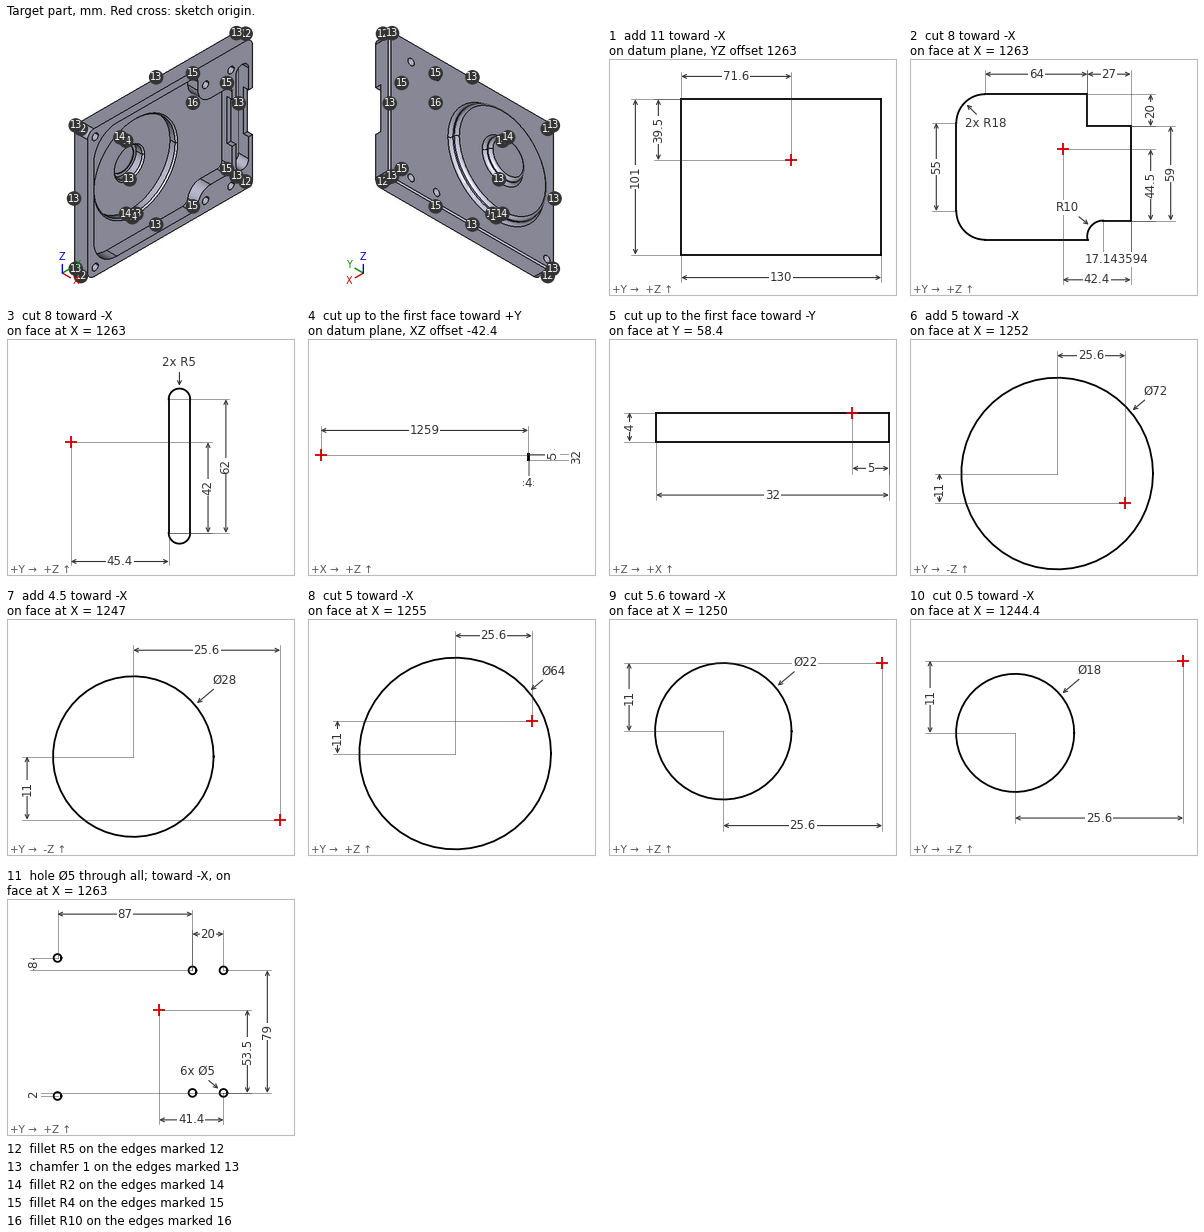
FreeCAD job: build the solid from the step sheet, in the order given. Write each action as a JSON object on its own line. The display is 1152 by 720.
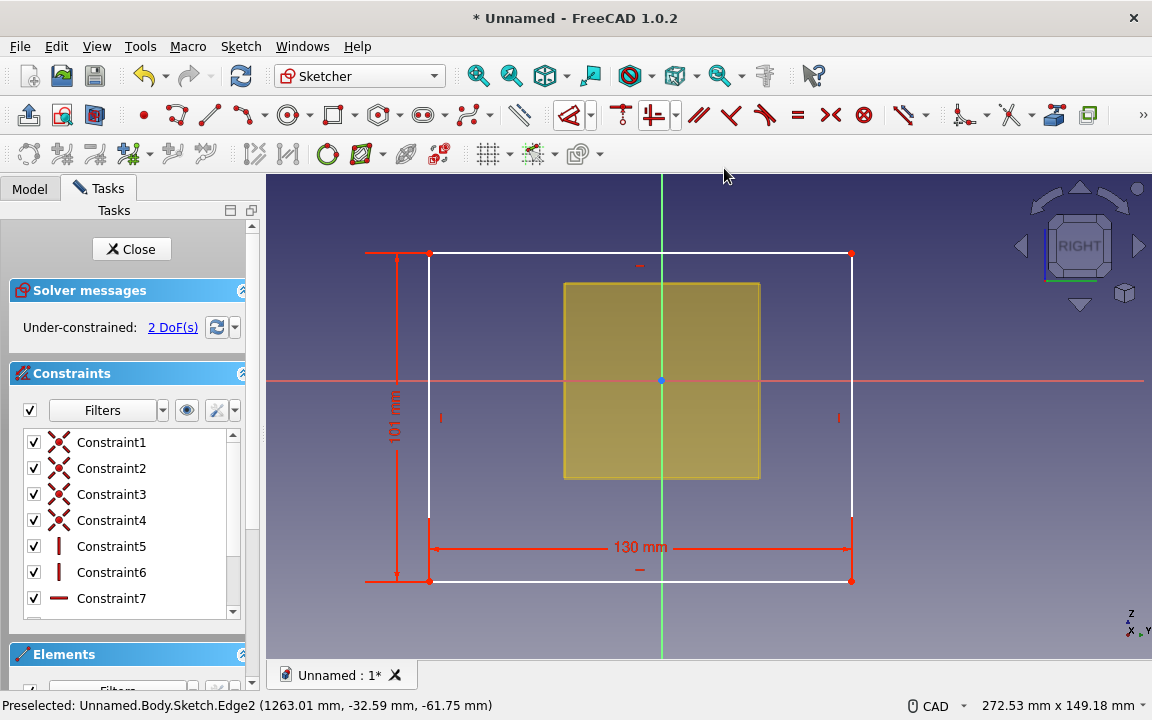
{"action": "left_click", "coordinate": [429, 253]}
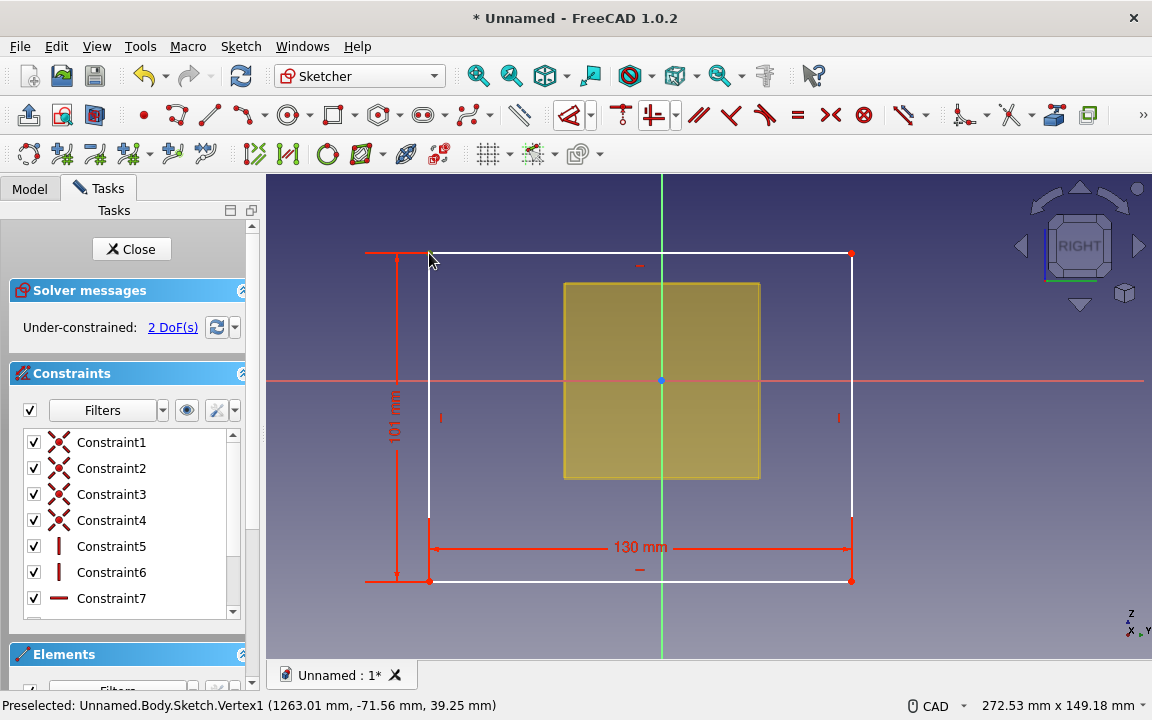
{"action": "key", "text": "l"}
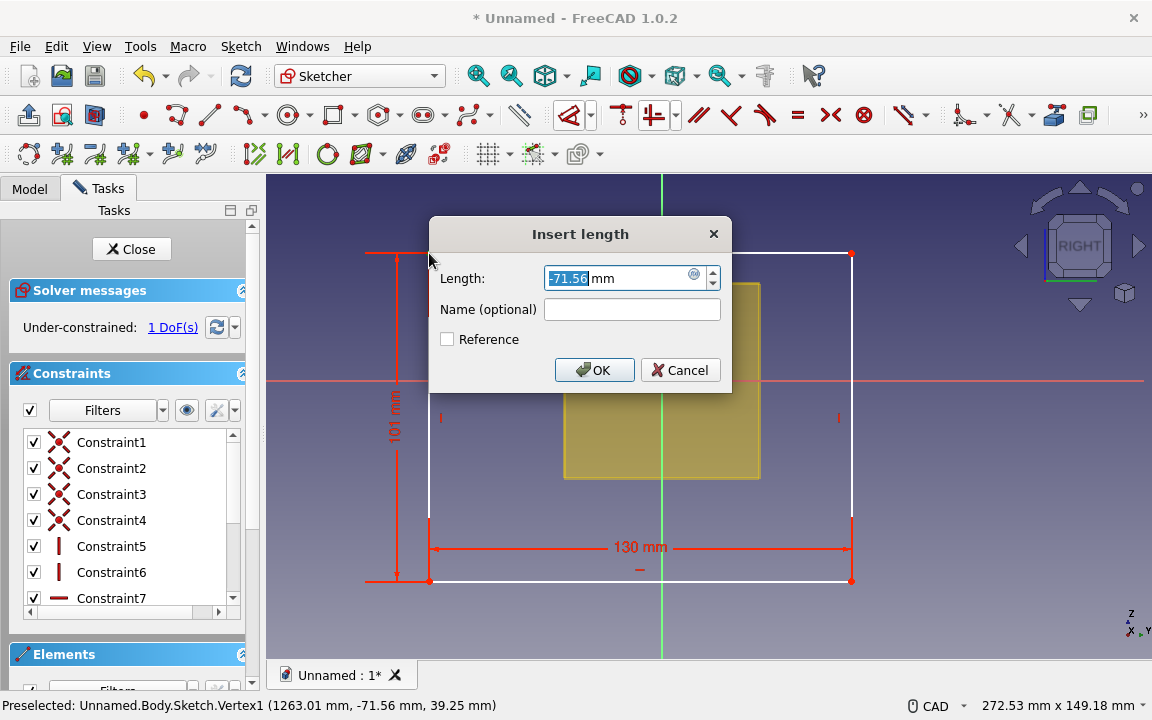
{"action": "type", "text": "-71.6"}
{"action": "key", "text": "Return"}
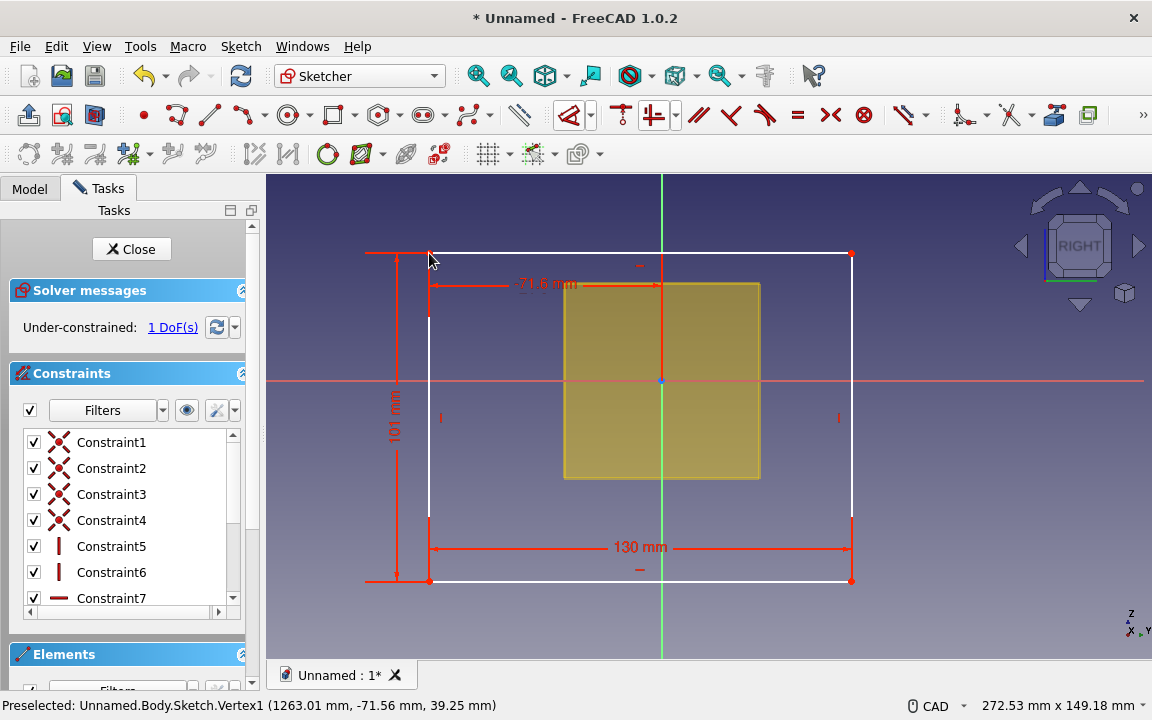
{"action": "left_click", "coordinate": [429, 253]}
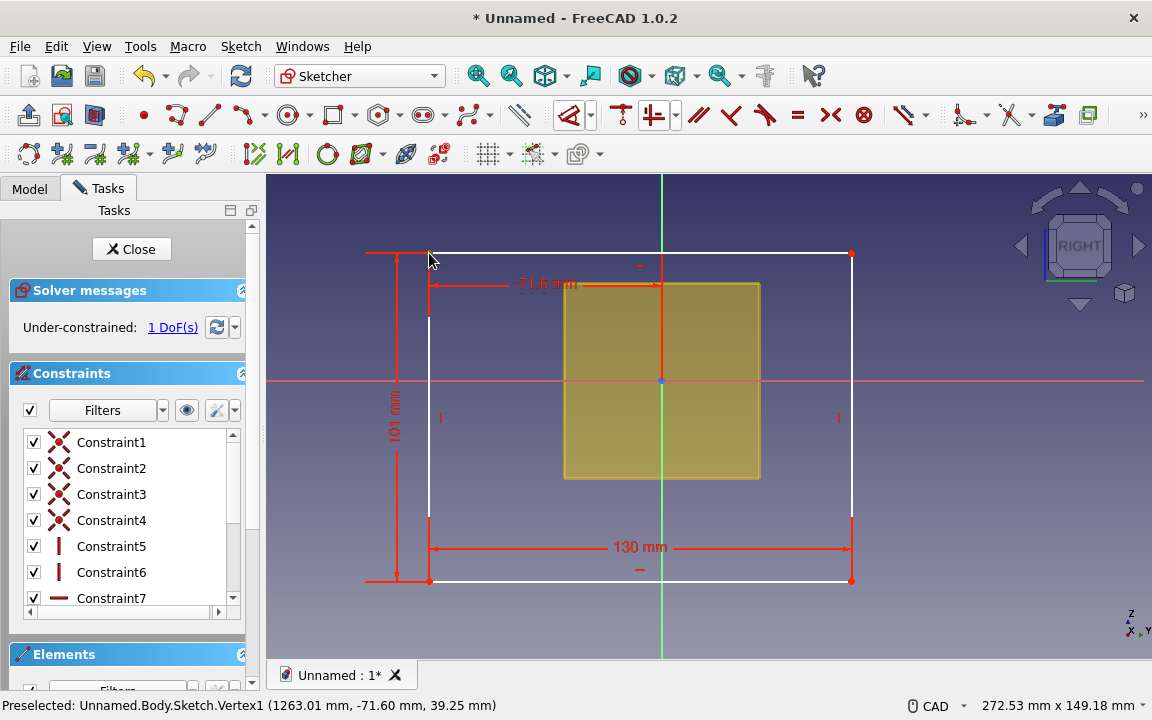
{"action": "key", "text": "i"}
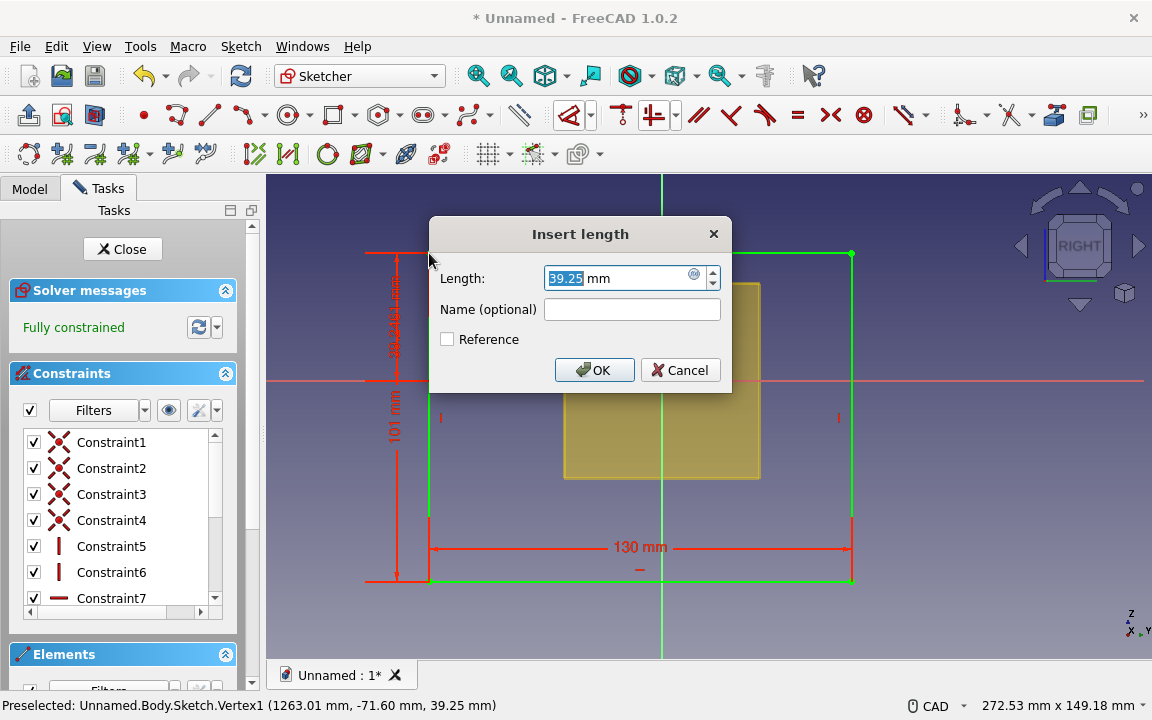
{"action": "type", "text": "39.5"}
{"action": "key", "text": "Return"}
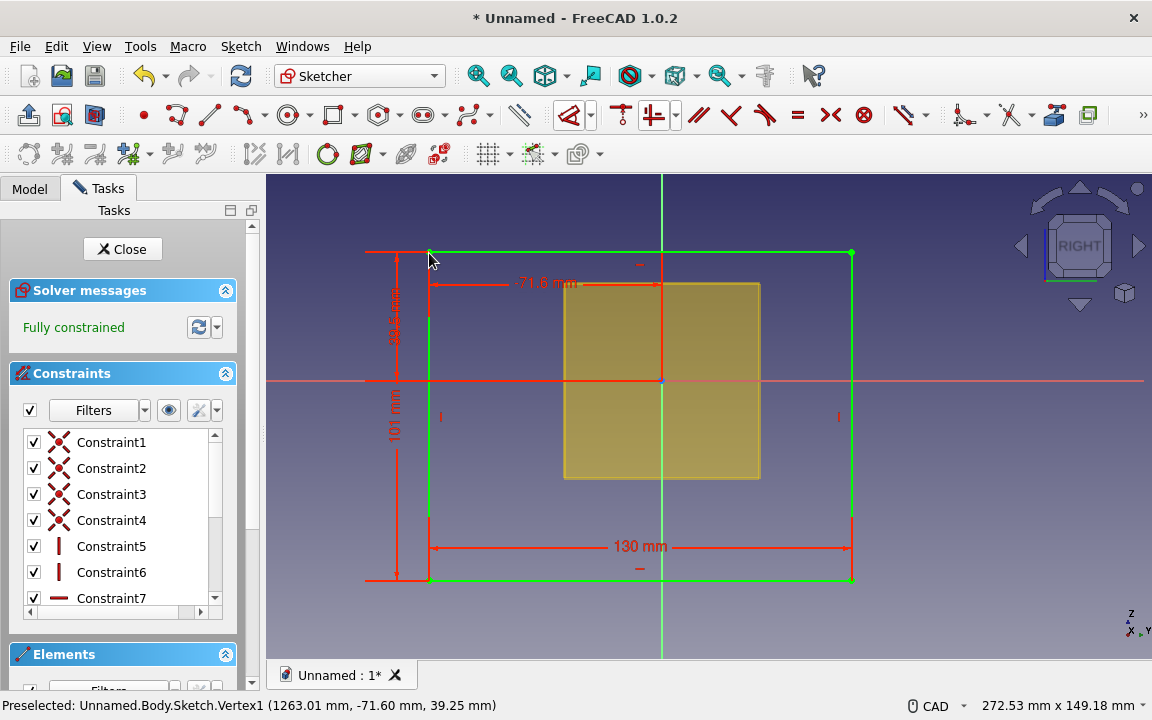
{"action": "left_click", "coordinate": [123, 249]}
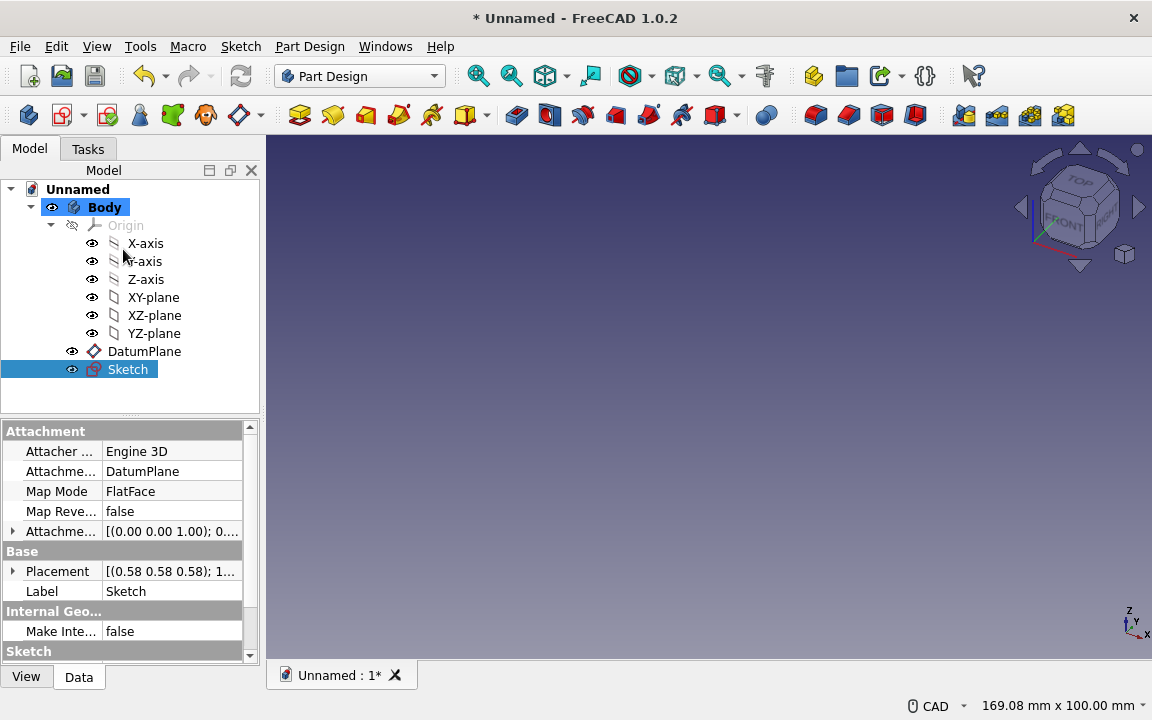
{"action": "left_click", "coordinate": [300, 116]}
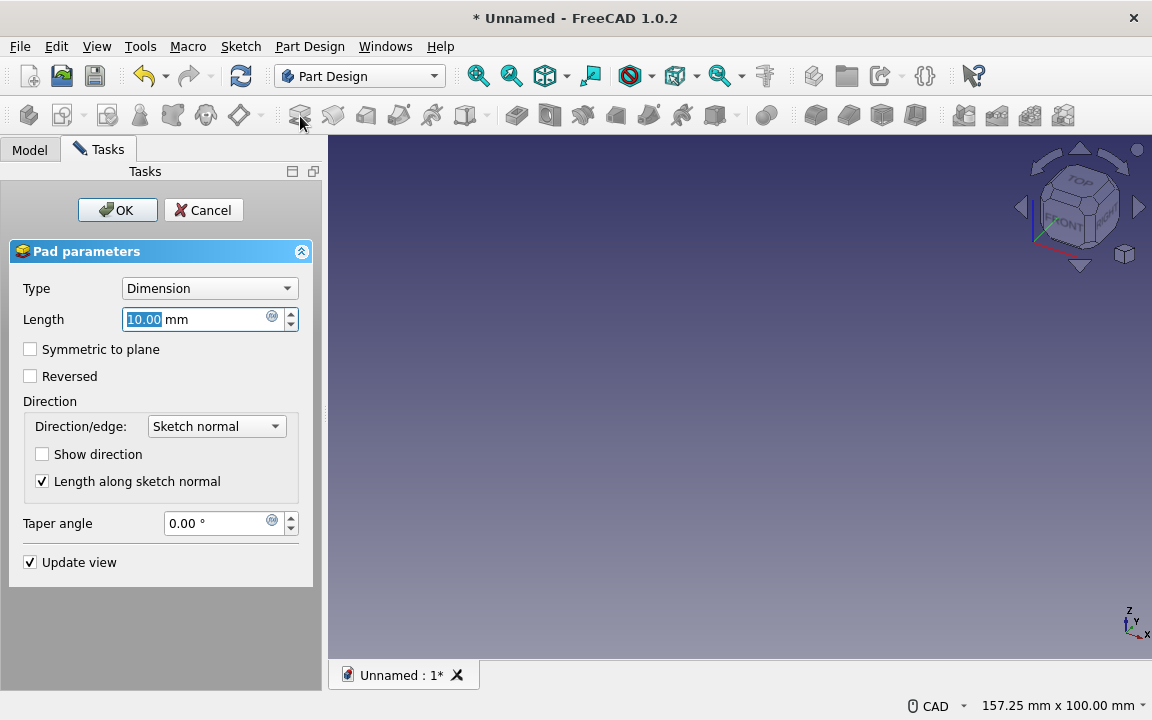
{"action": "type", "text": "11"}
{"action": "key", "text": "Tab"}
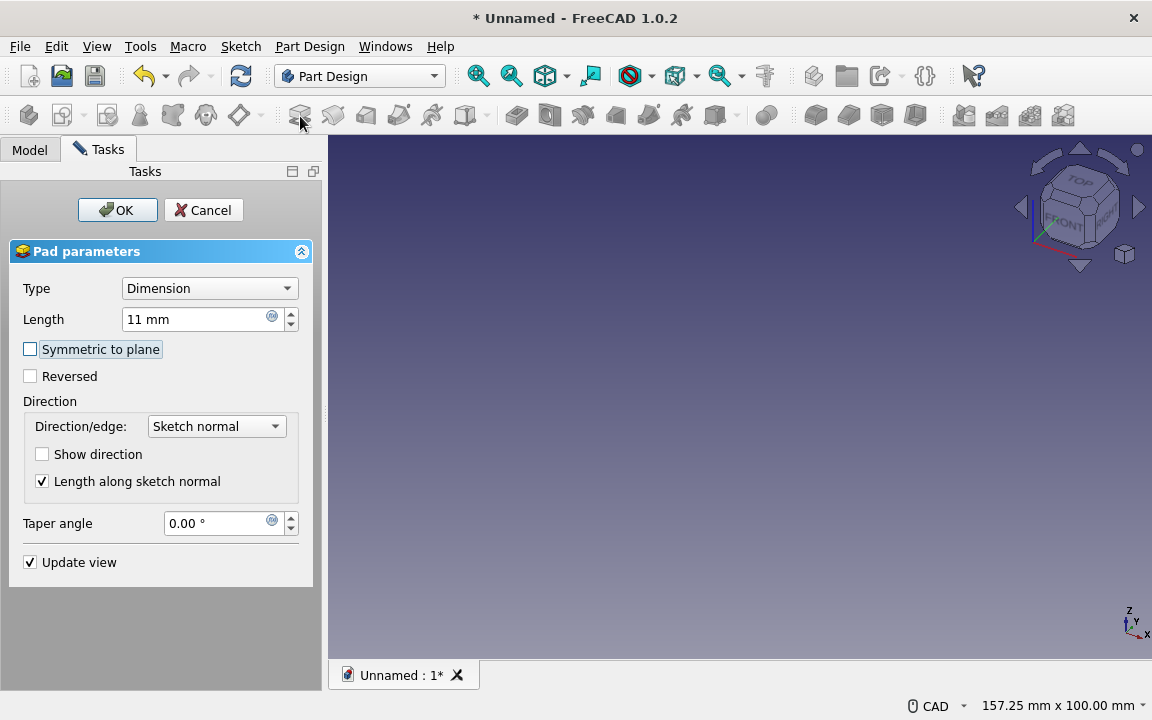
{"action": "left_click", "coordinate": [31, 376]}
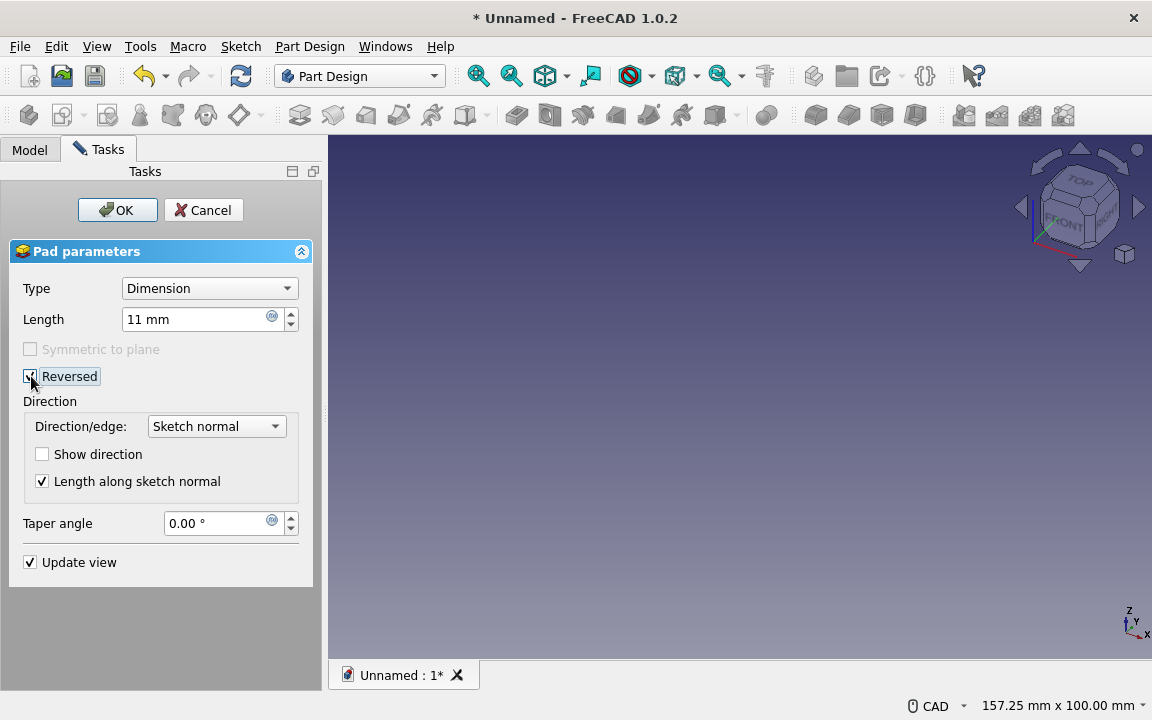
{"action": "left_click", "coordinate": [118, 210]}